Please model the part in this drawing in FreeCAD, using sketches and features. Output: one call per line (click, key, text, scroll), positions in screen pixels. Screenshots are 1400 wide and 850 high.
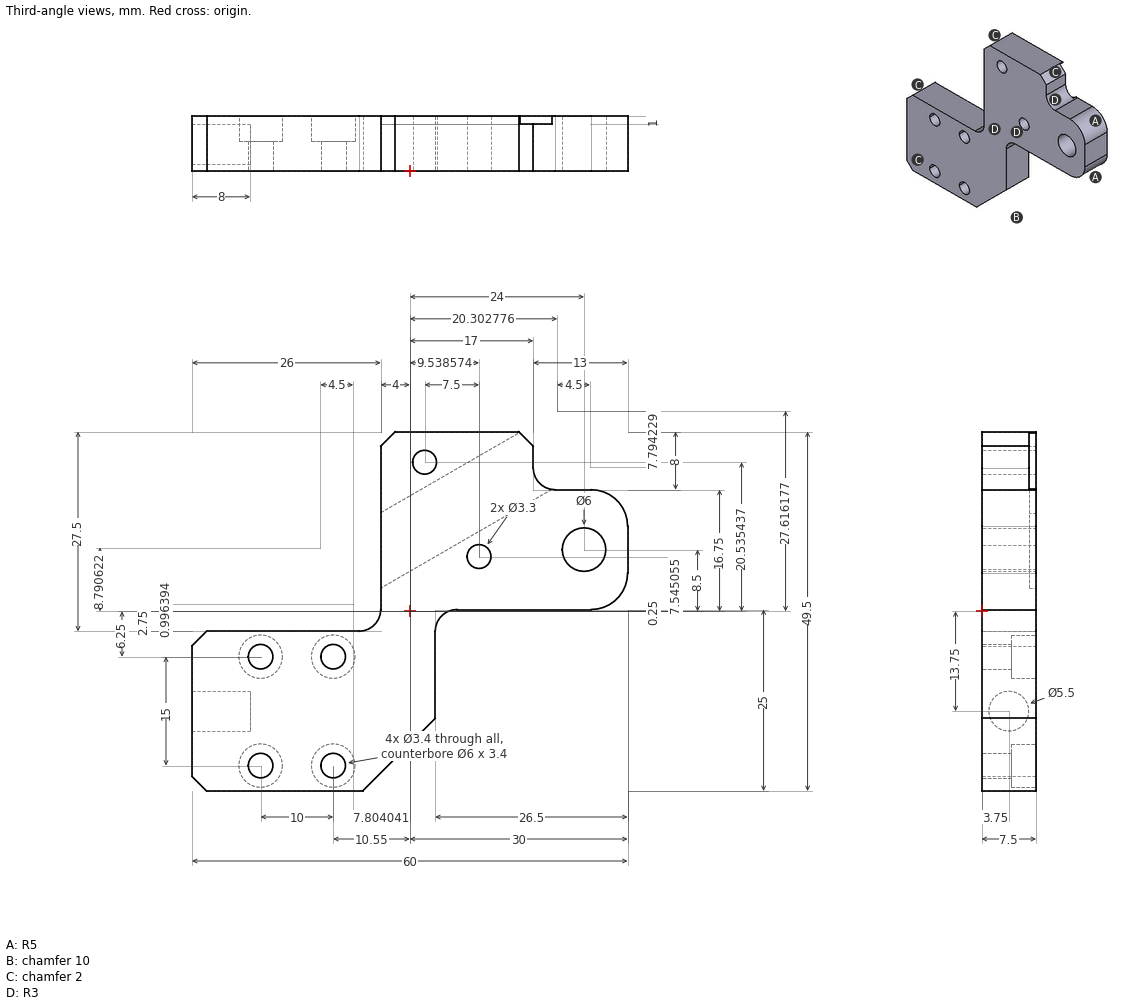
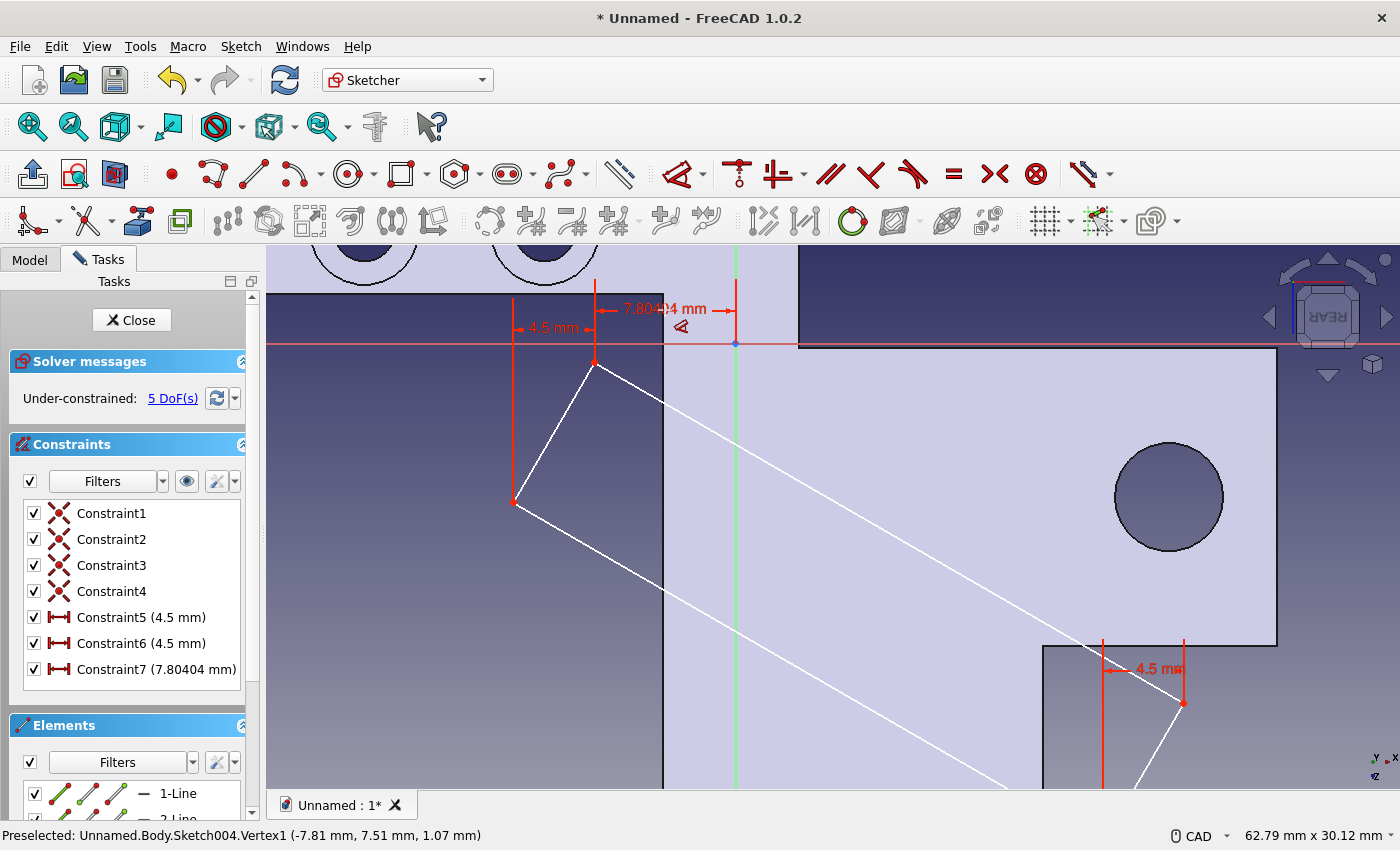
scroll(595, 363, up, 4)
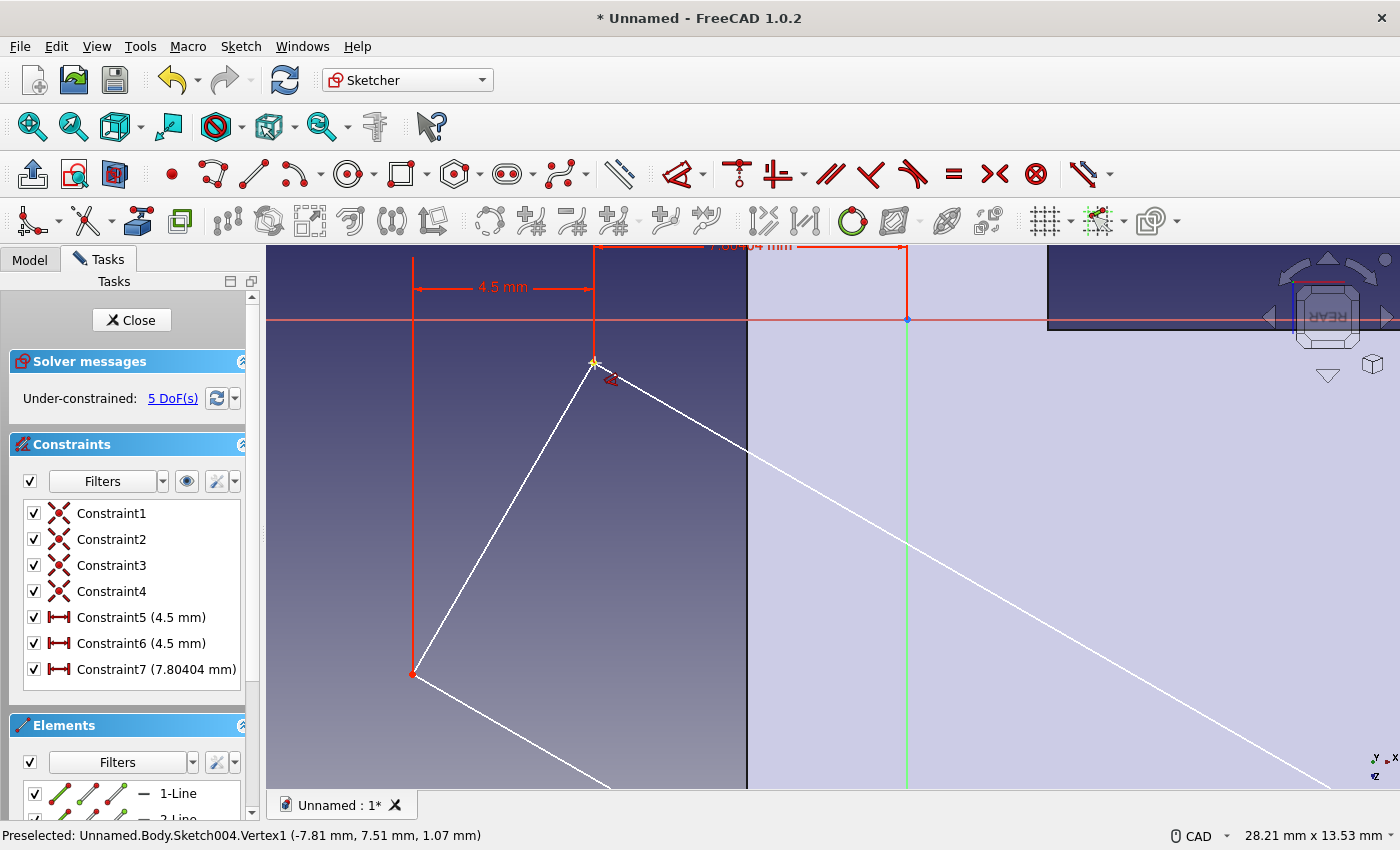
click(594, 363)
click(560, 341)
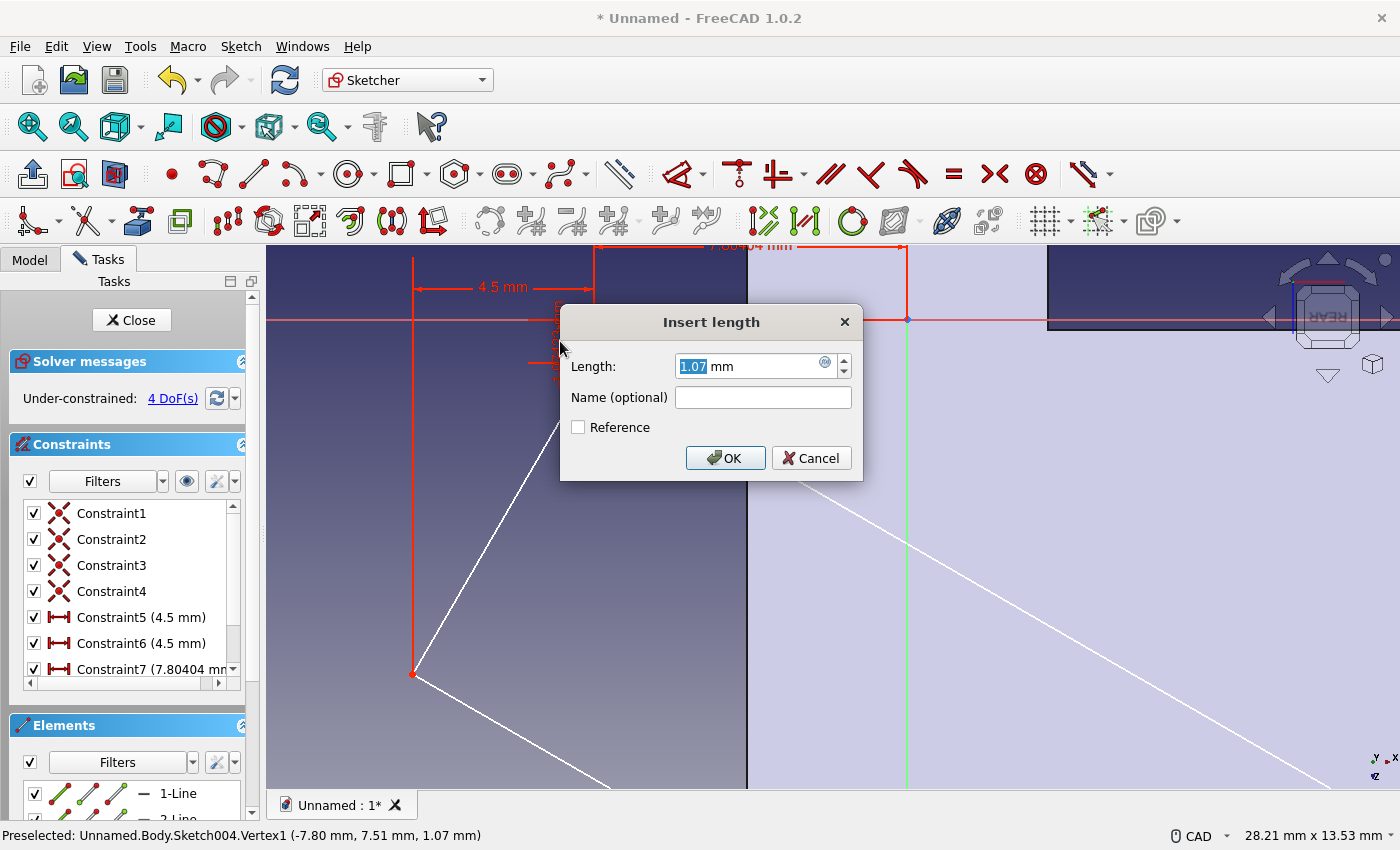
text(0.996394)
key(Return)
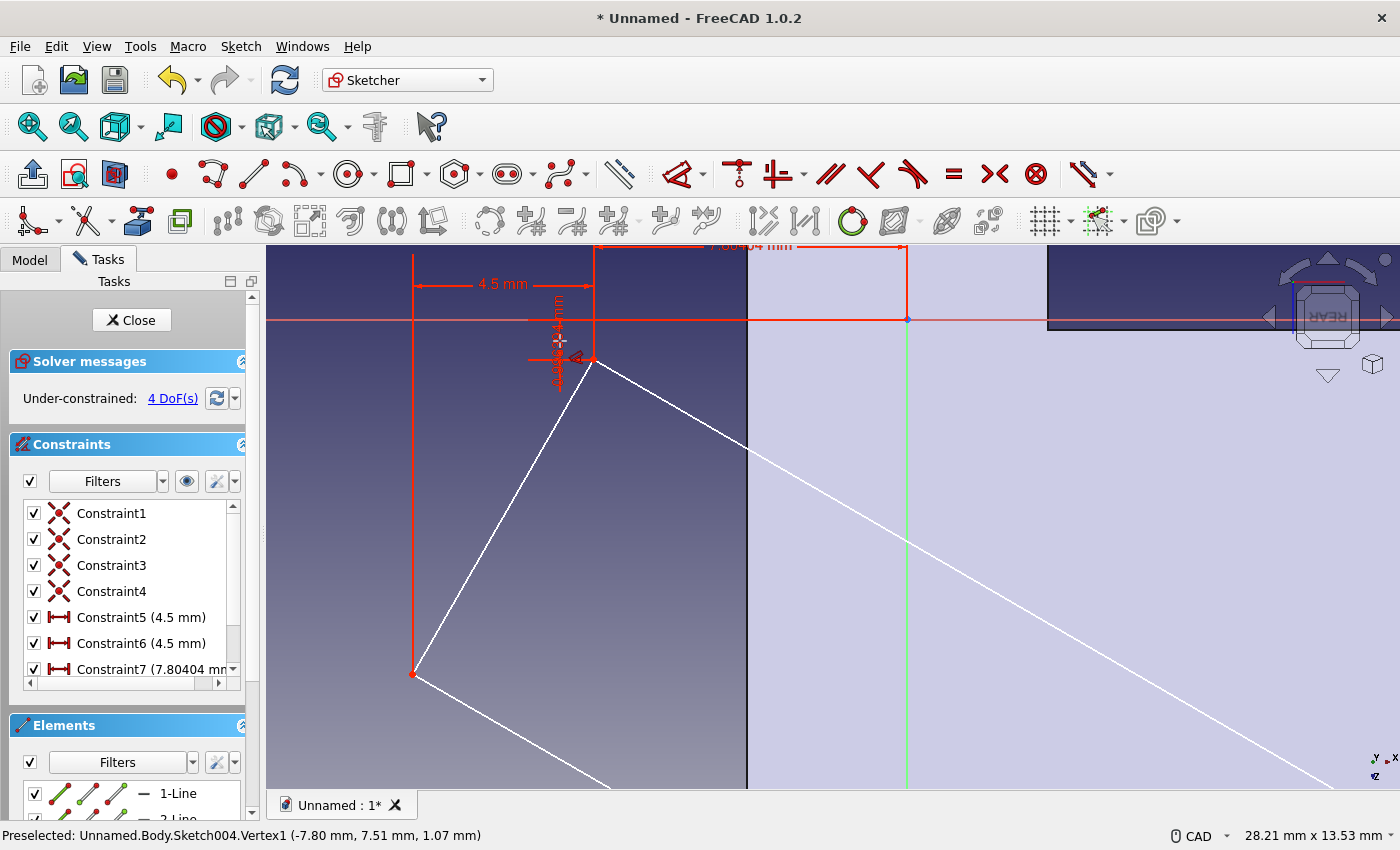
click(413, 674)
click(379, 497)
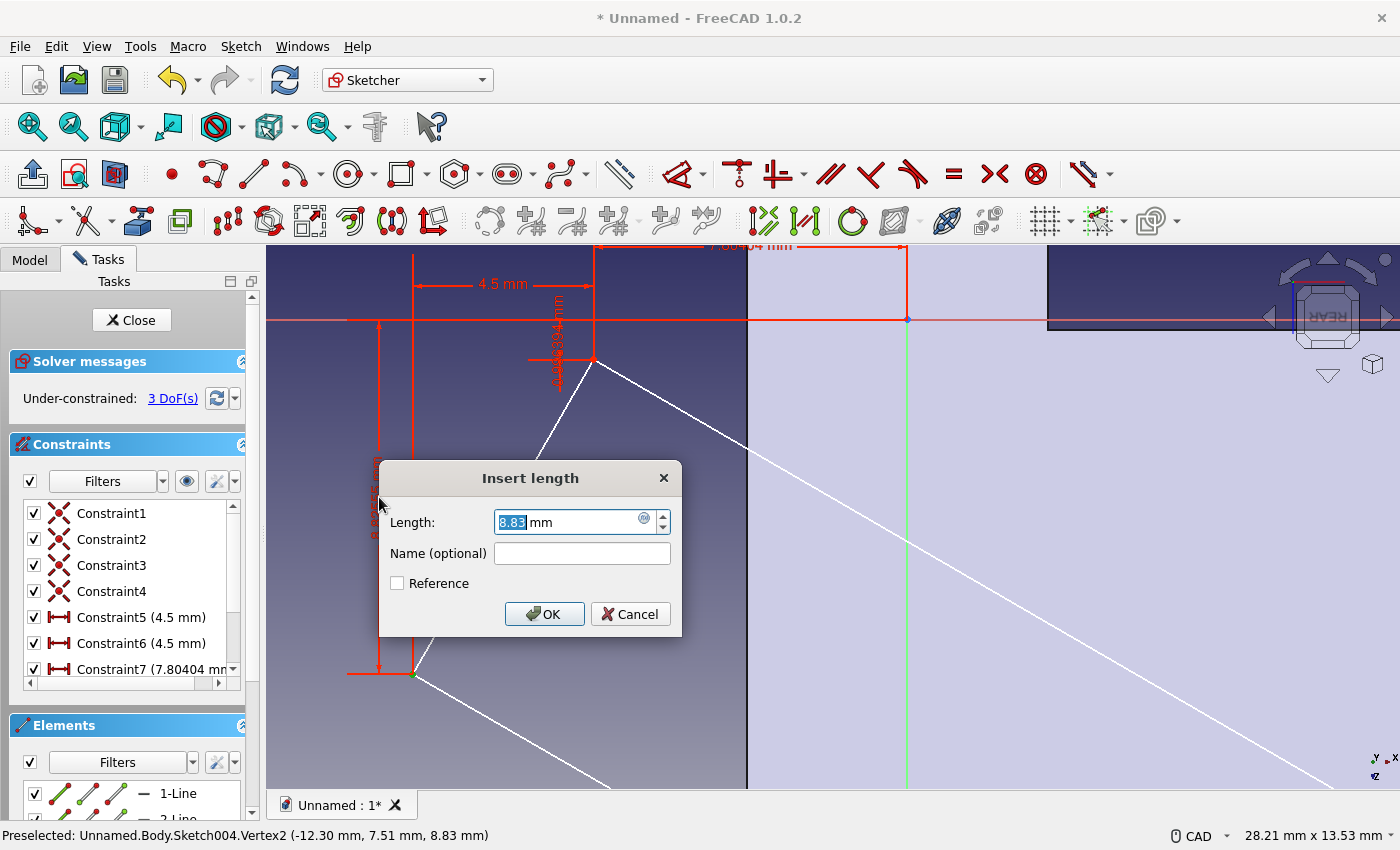
text(8.790622)
key(Return)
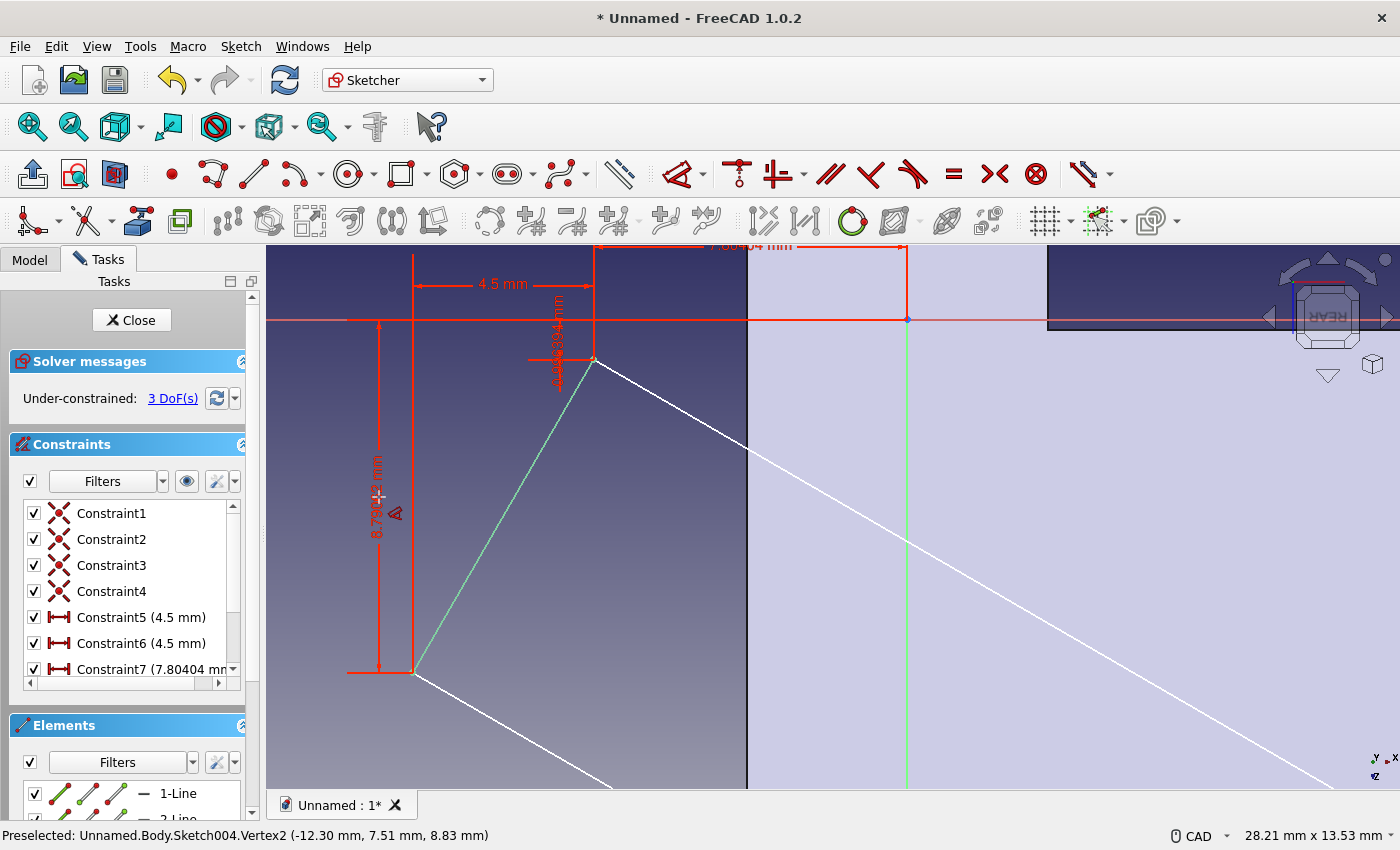
scroll(595, 363, down, 6)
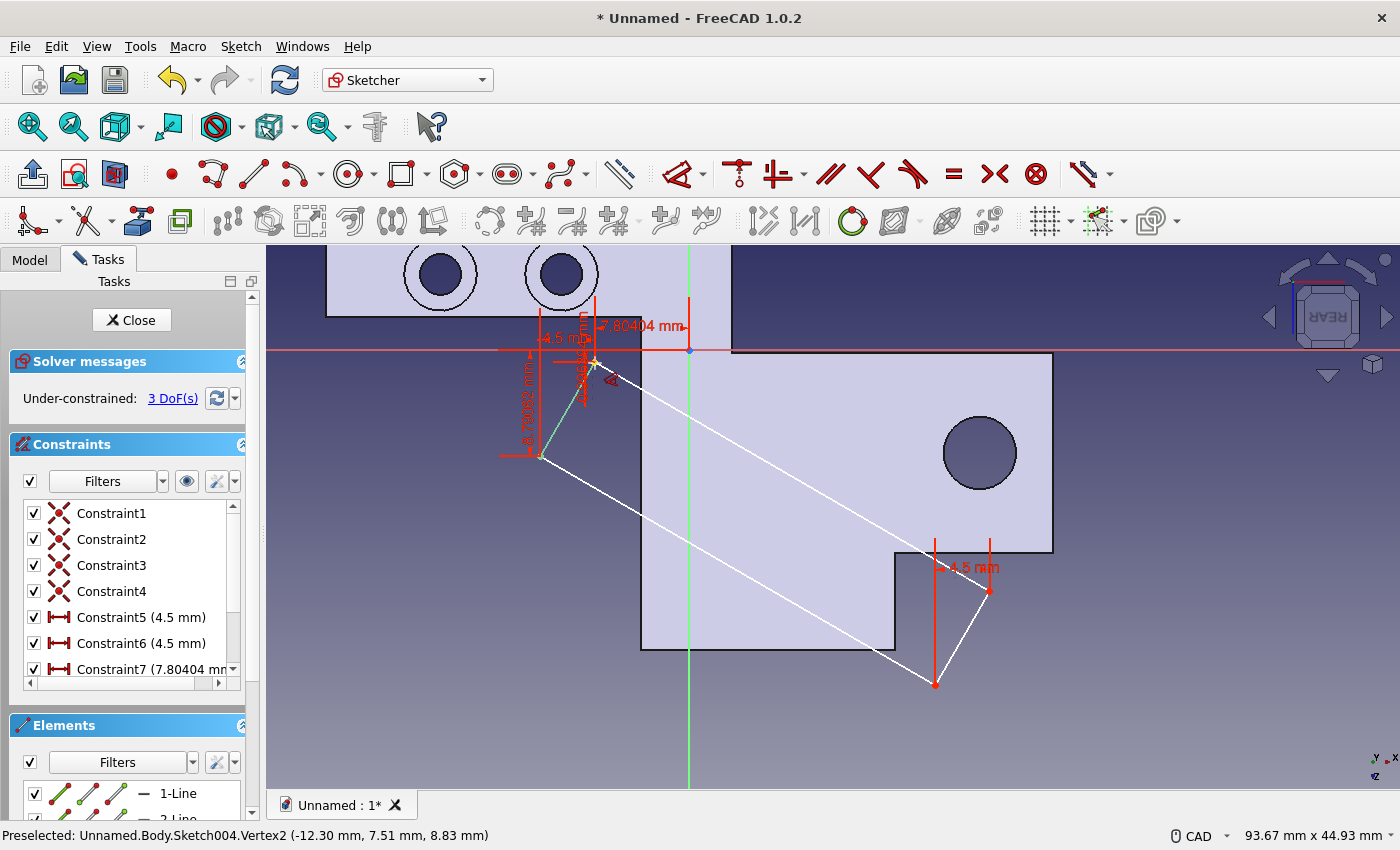
click(952, 657)
click(1024, 638)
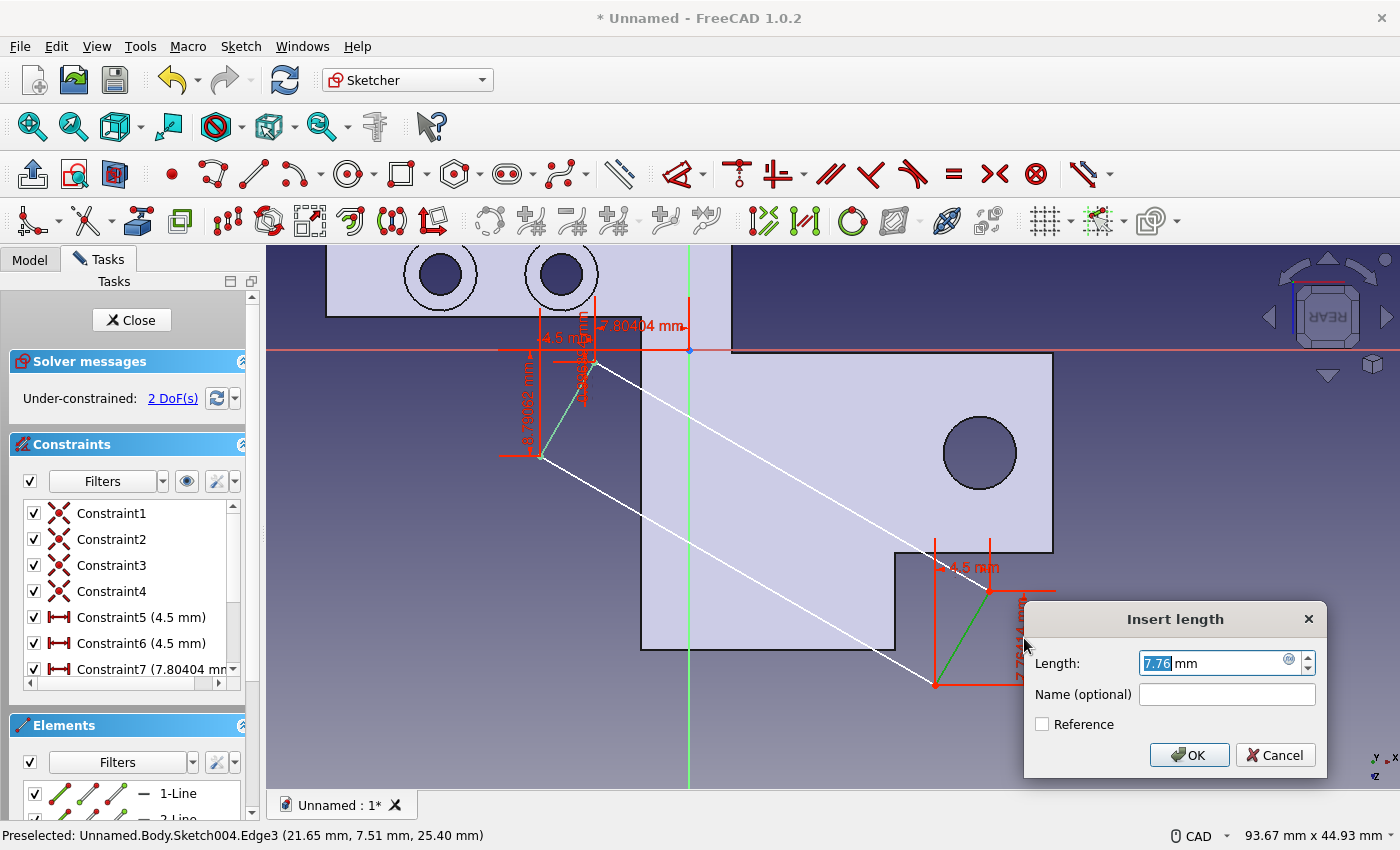
text(7.794229)
key(Return)